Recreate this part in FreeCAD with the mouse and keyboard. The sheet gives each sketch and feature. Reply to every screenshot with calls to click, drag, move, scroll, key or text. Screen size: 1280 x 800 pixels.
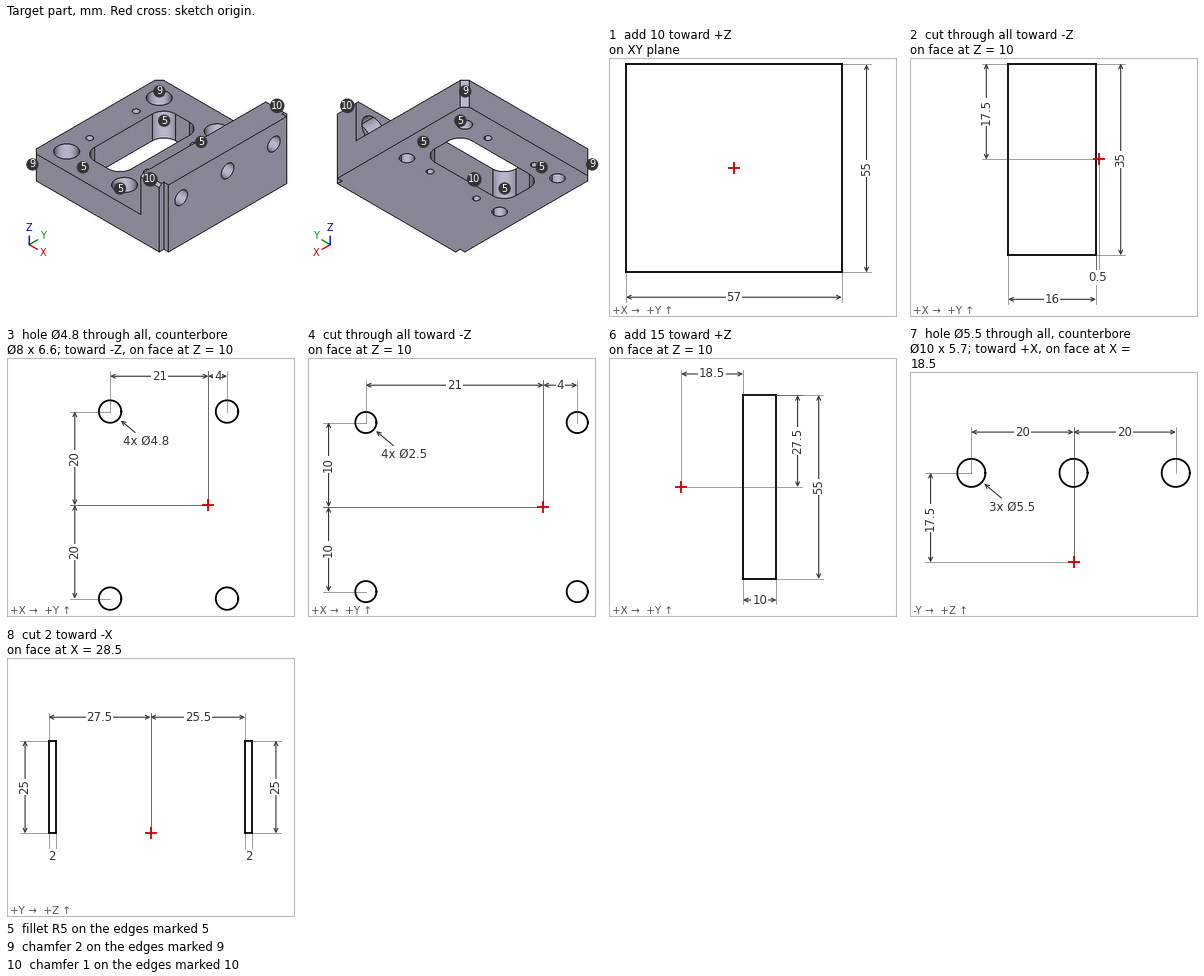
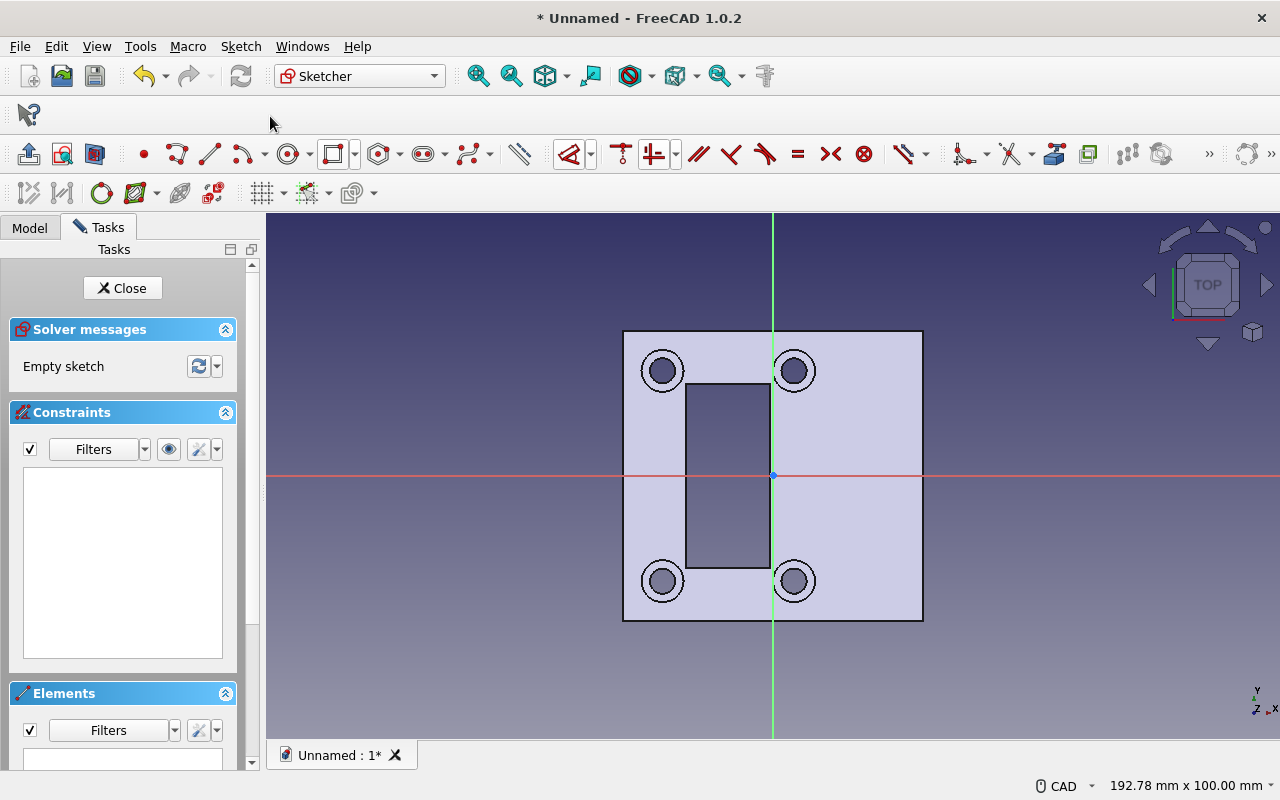
scroll(742, 476, up, 5)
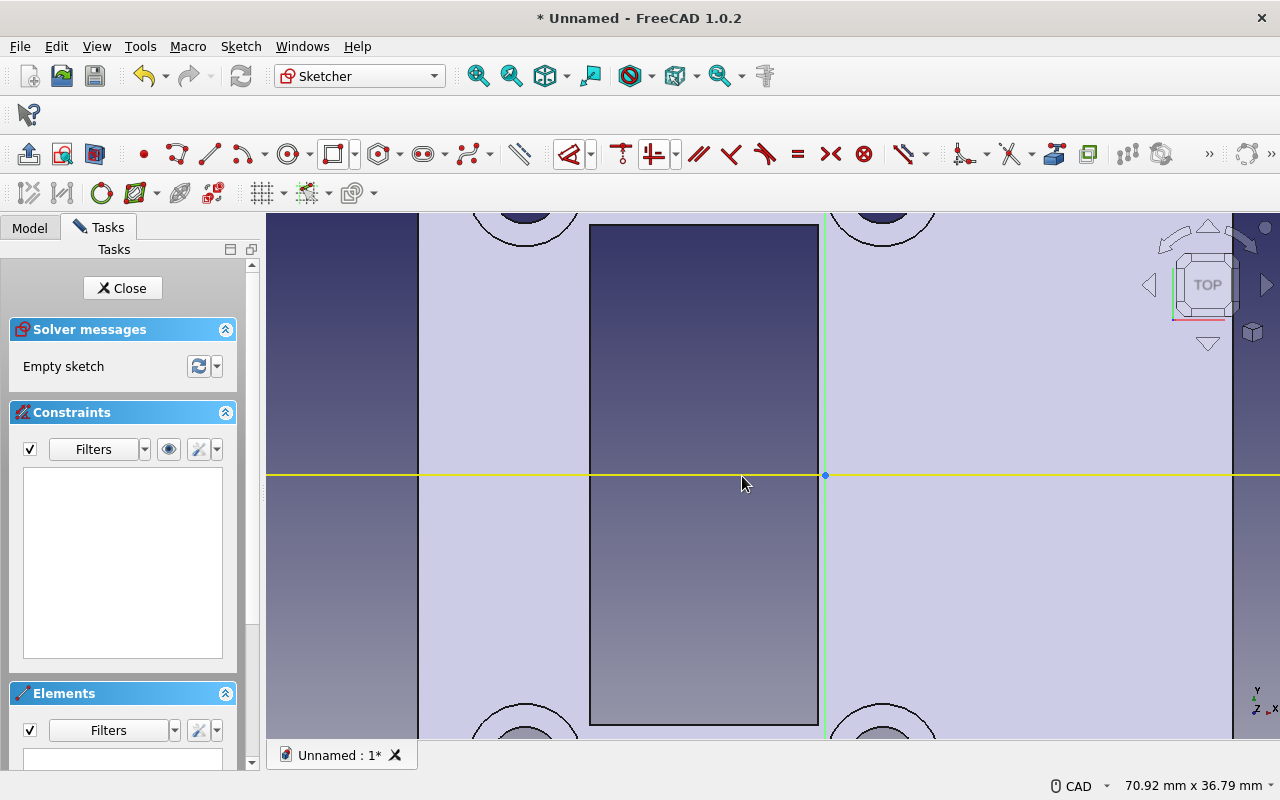
key(g)
key(c)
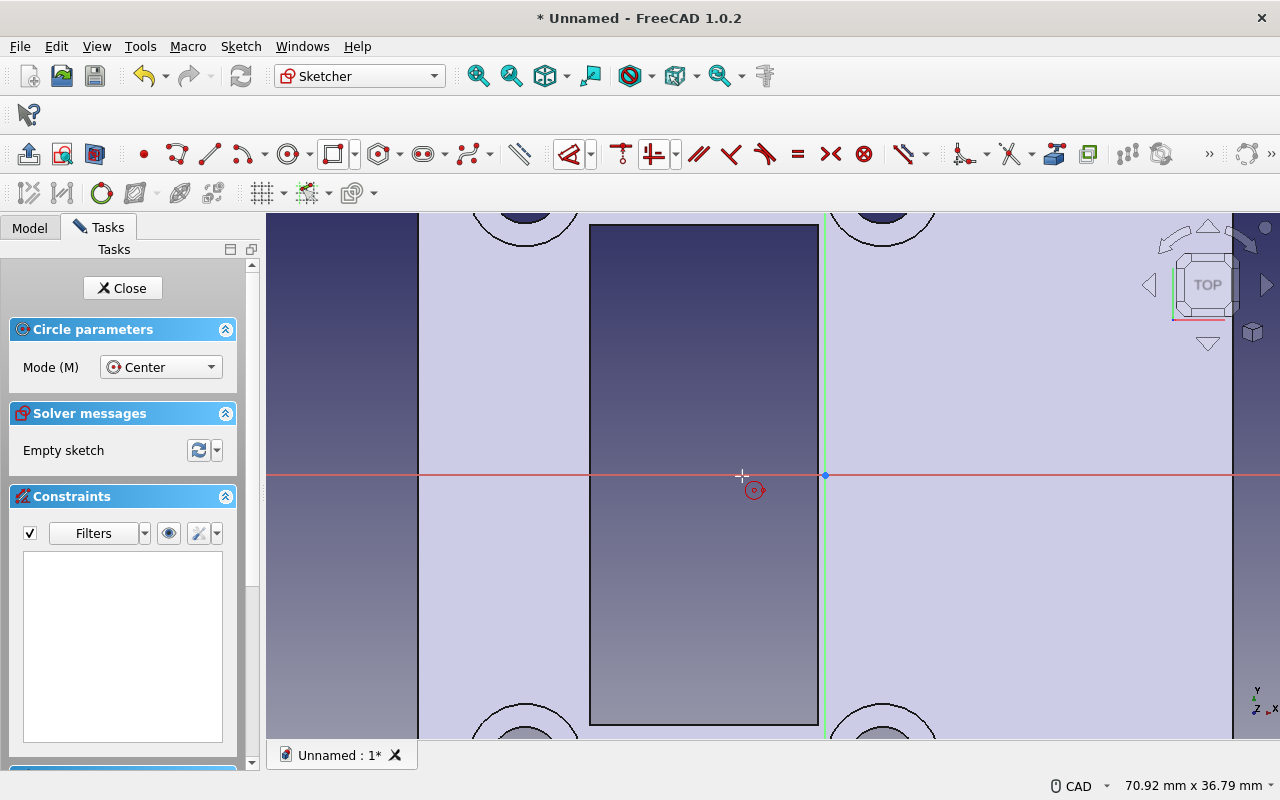
scroll(525, 332, up, 2)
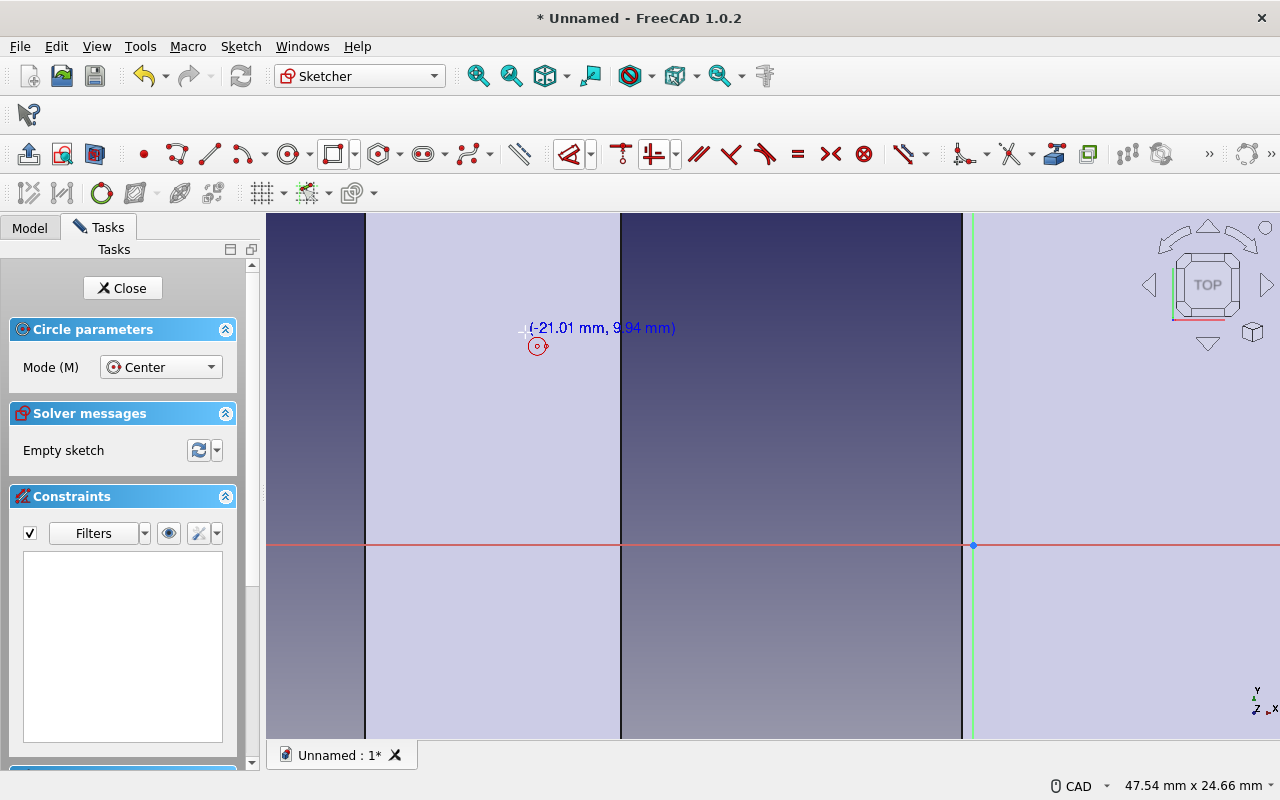
click(525, 332)
move(544, 313)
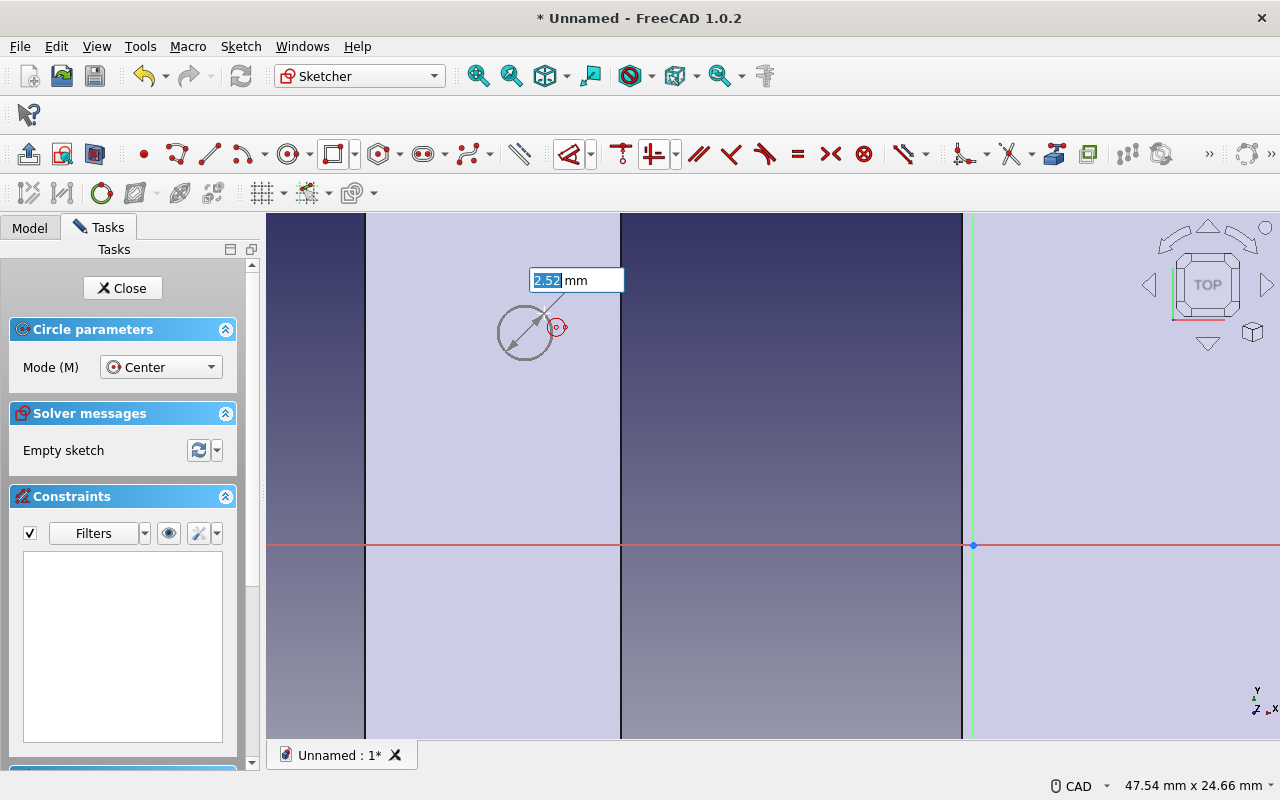
text(2.5)
key(Return)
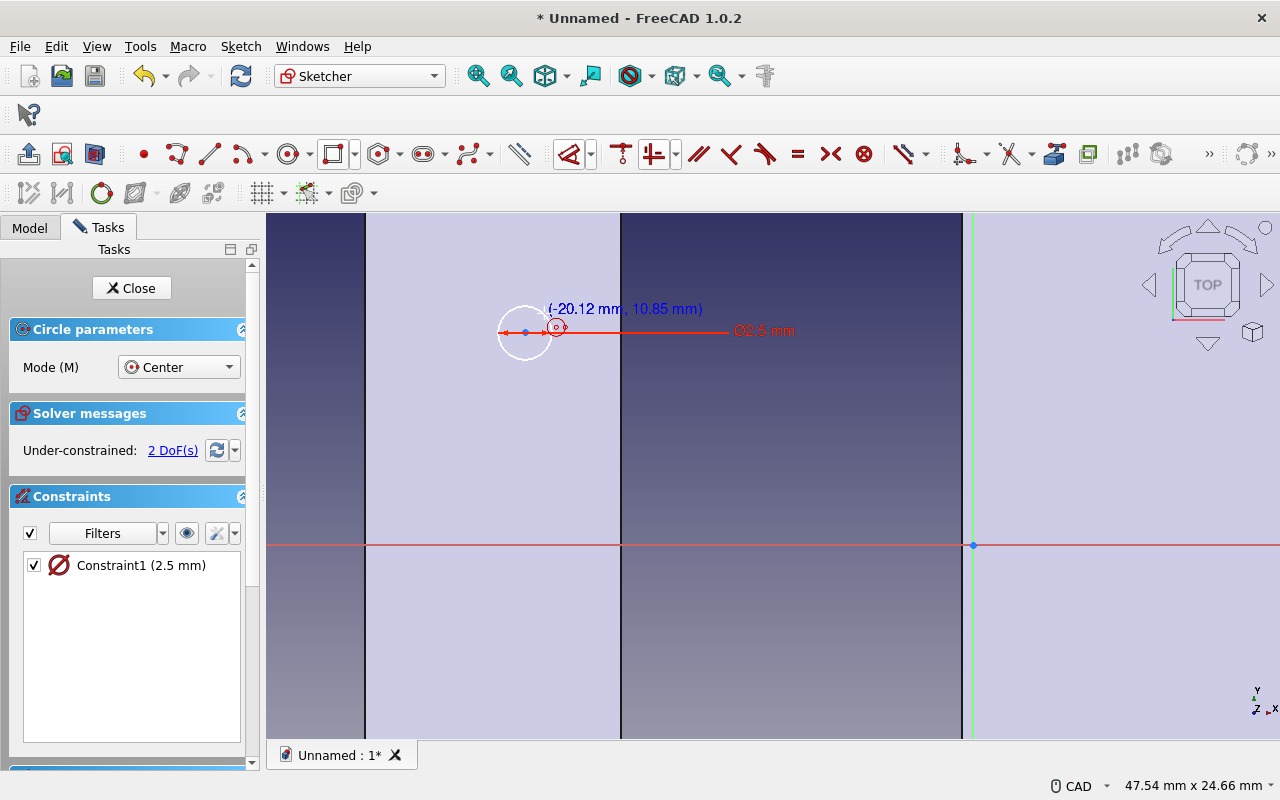
scroll(527, 335, down, 2)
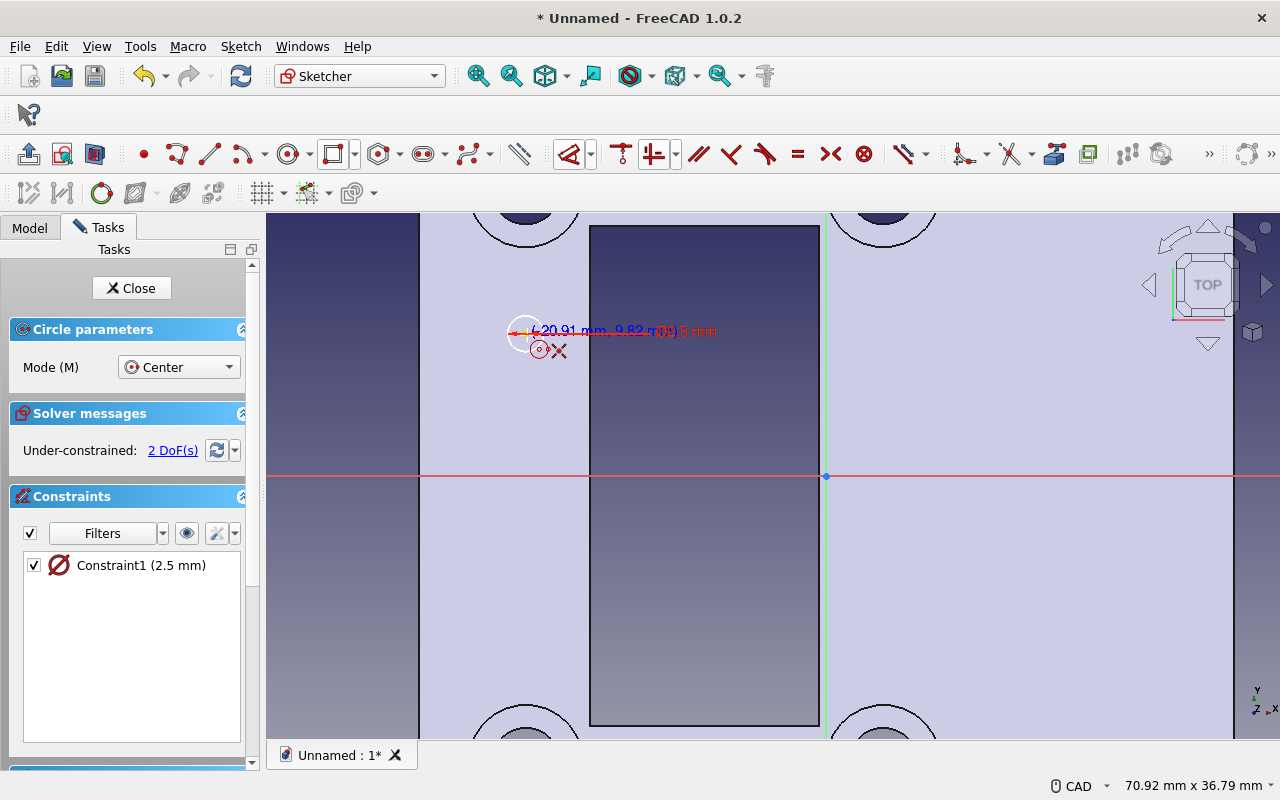
scroll(526, 619, up, 2)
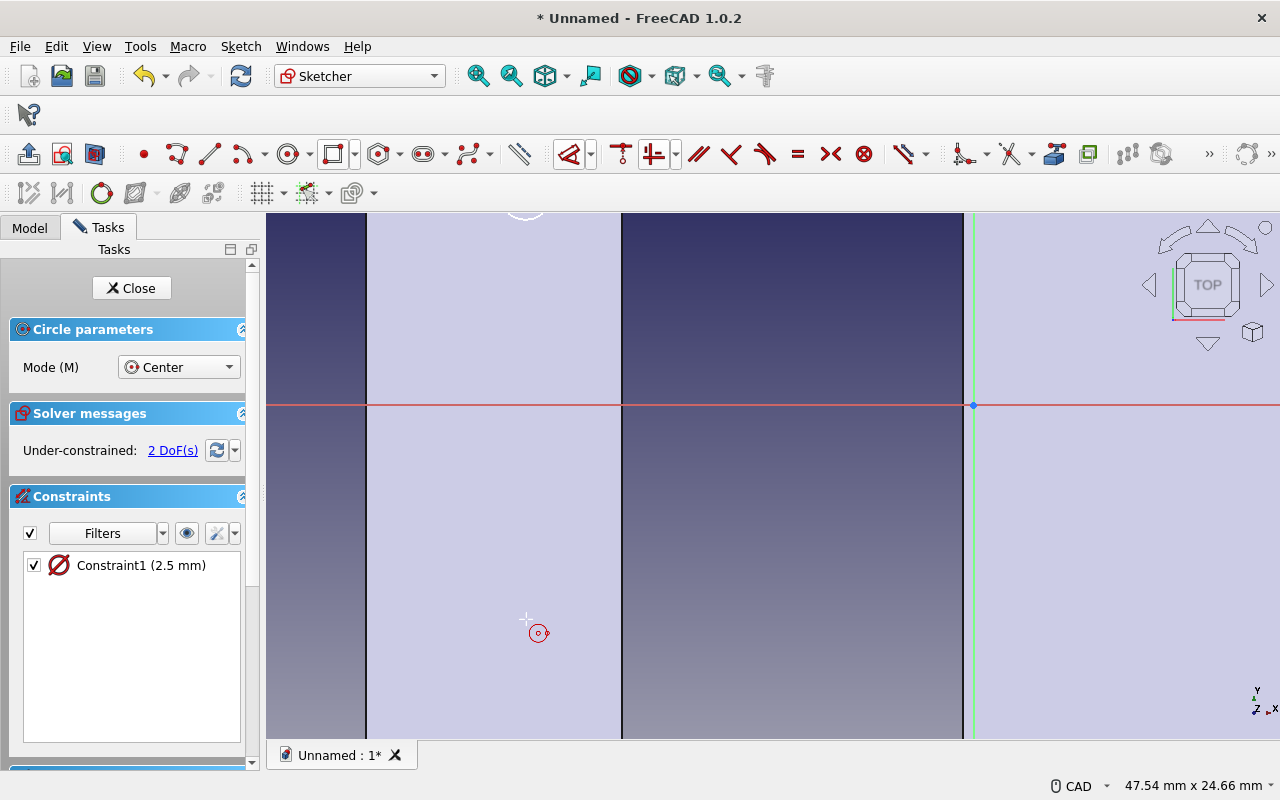
click(526, 619)
move(545, 600)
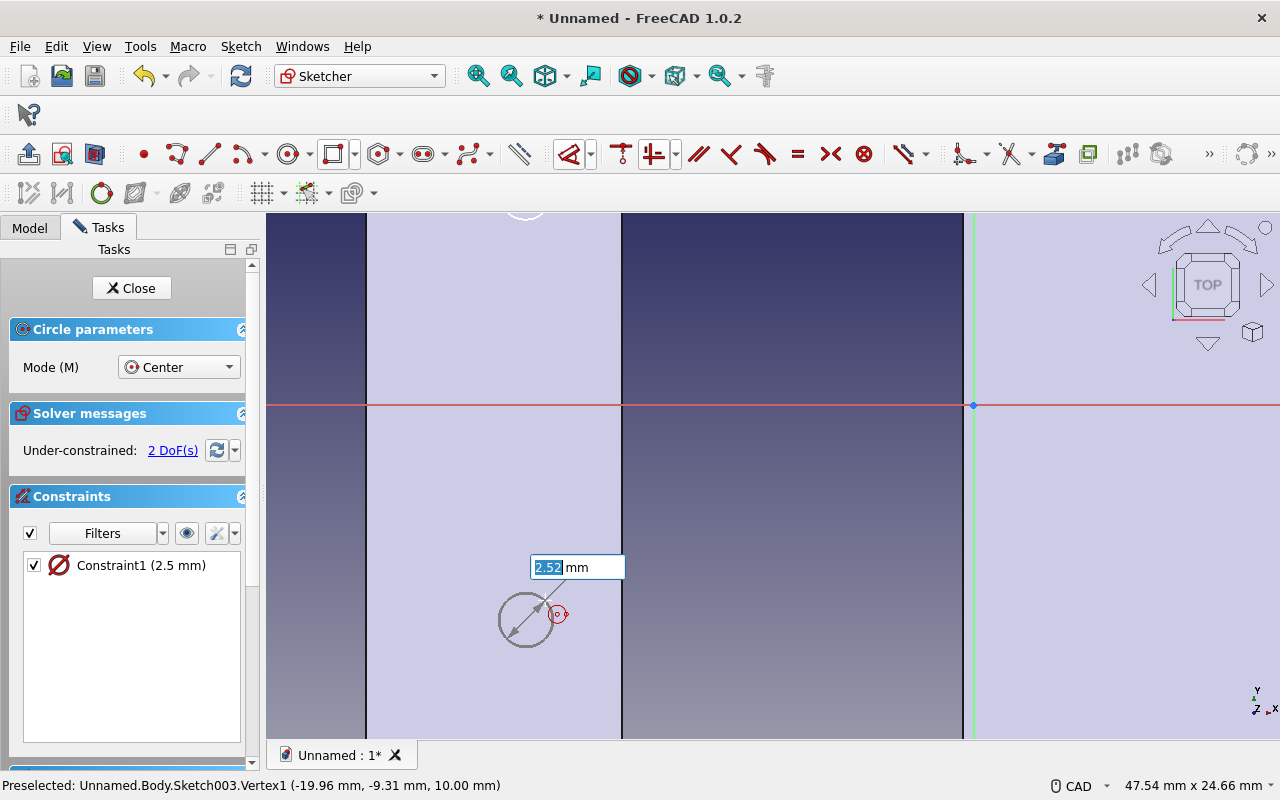
text(2.5)
key(Return)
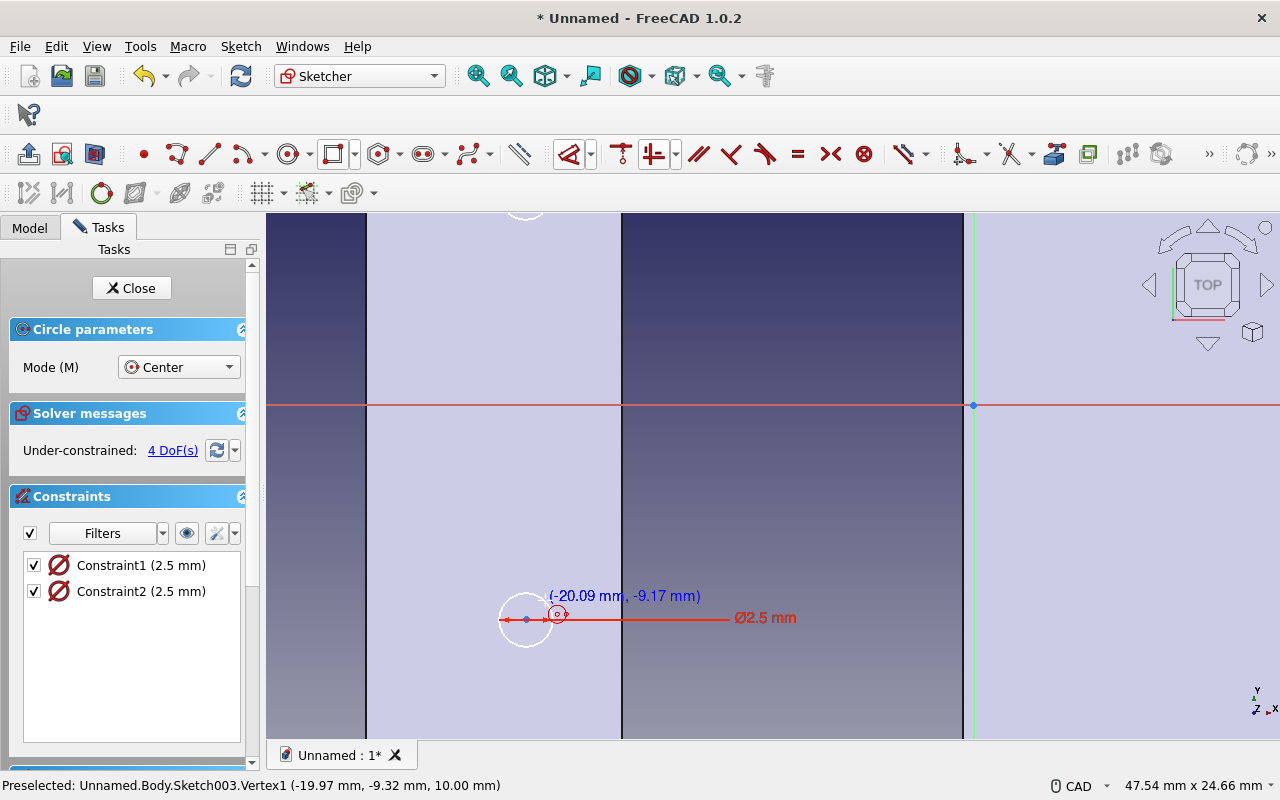
scroll(526, 619, down, 2)